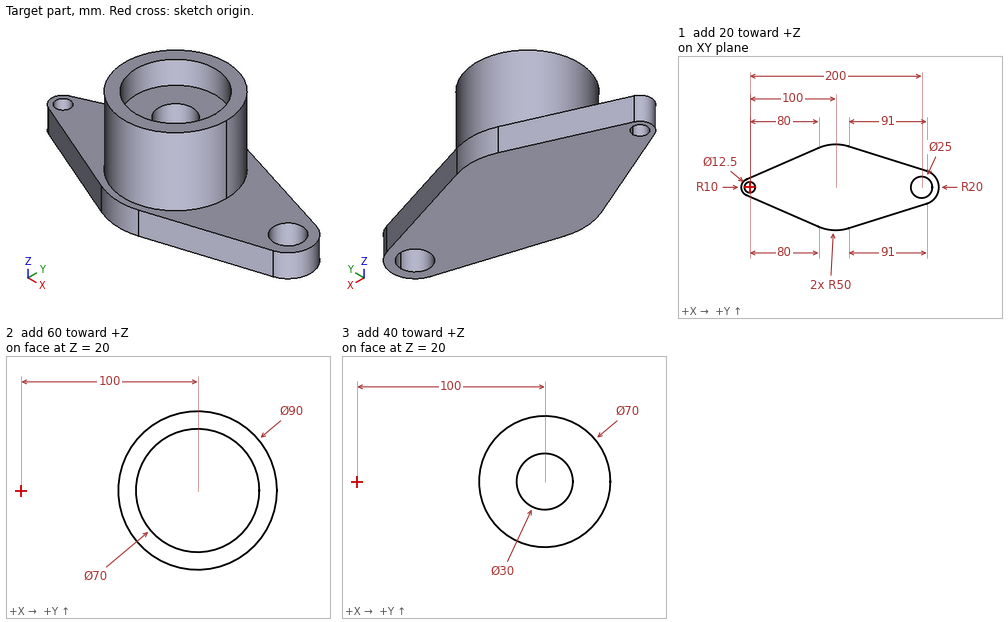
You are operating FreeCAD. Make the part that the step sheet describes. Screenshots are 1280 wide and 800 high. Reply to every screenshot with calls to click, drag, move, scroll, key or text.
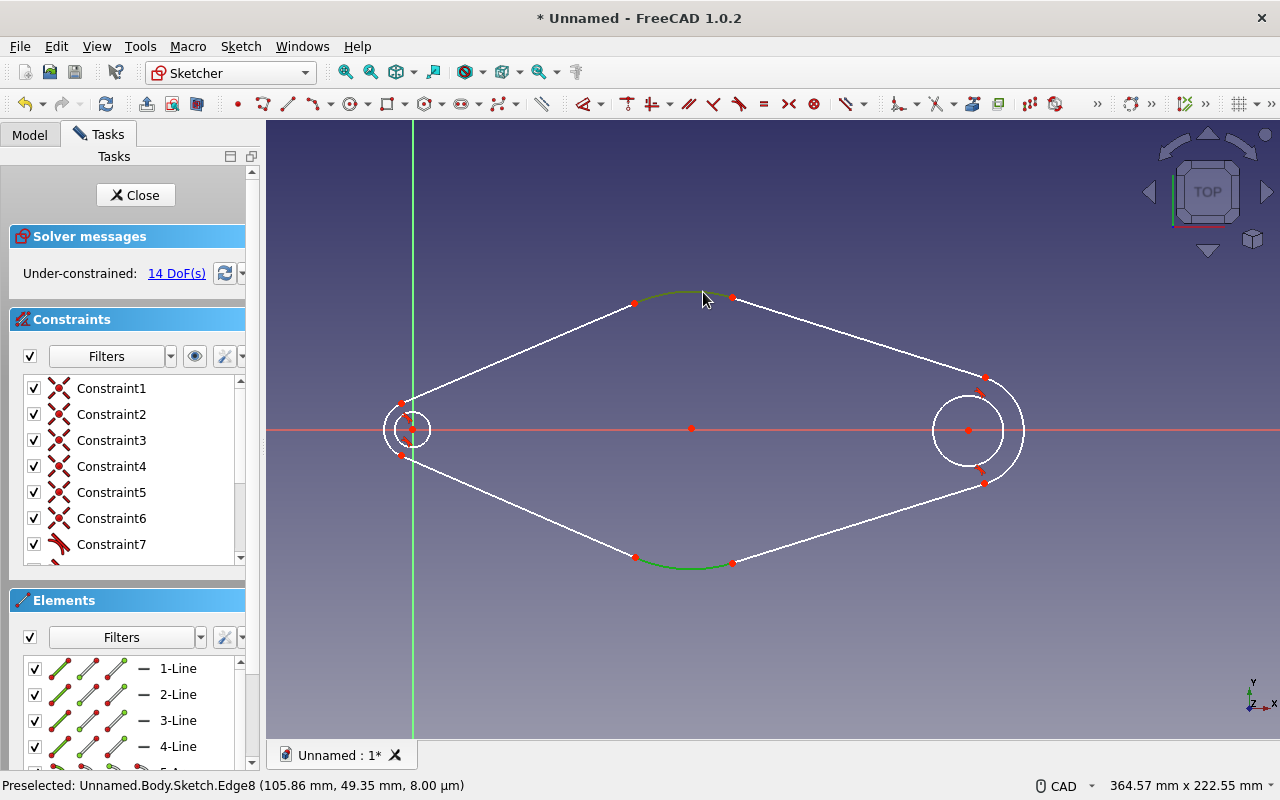
click(764, 104)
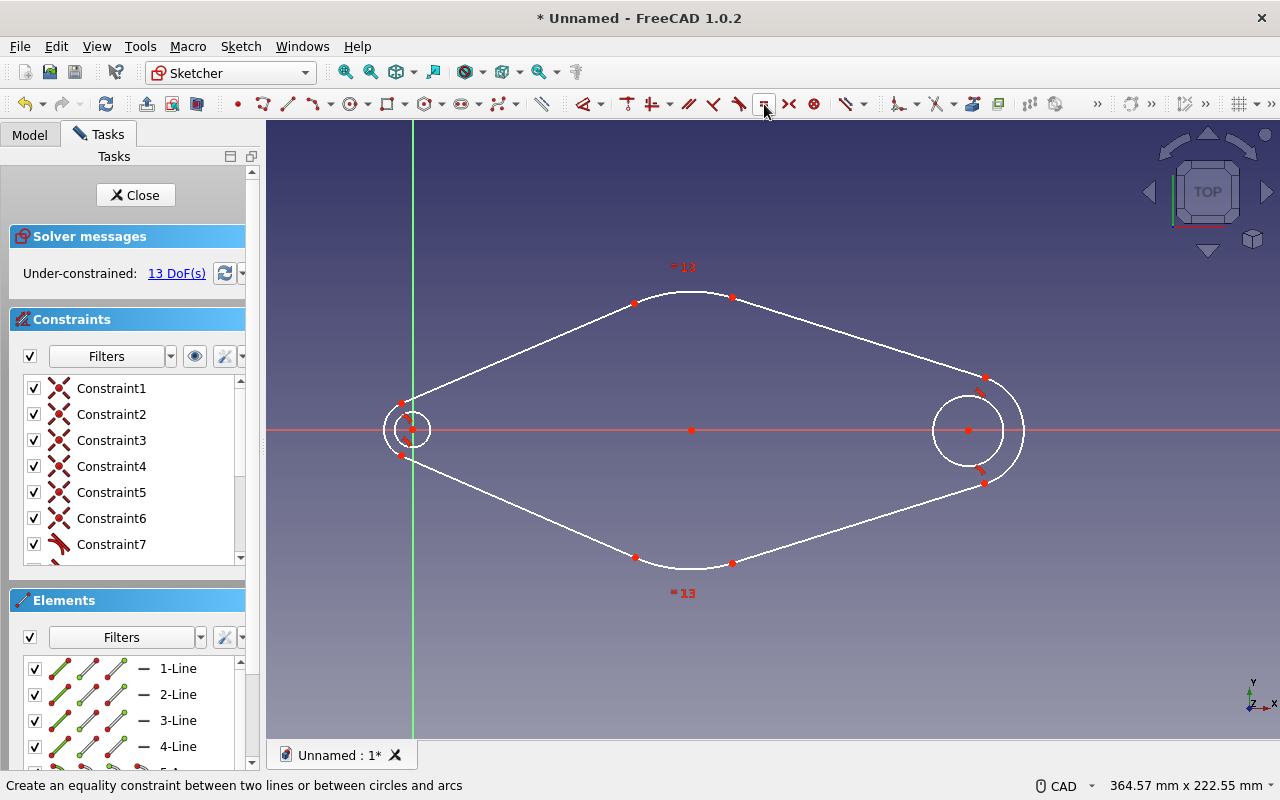
click(691, 431)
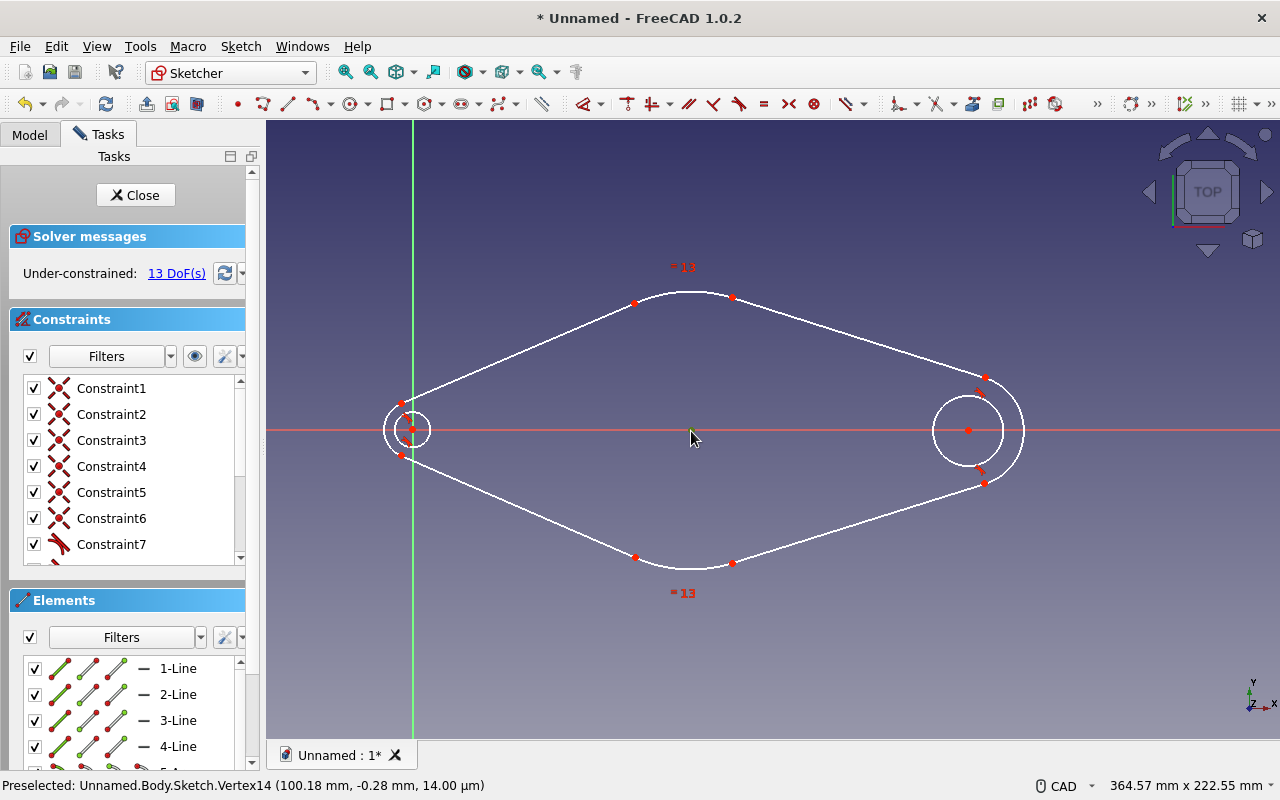
click(353, 430)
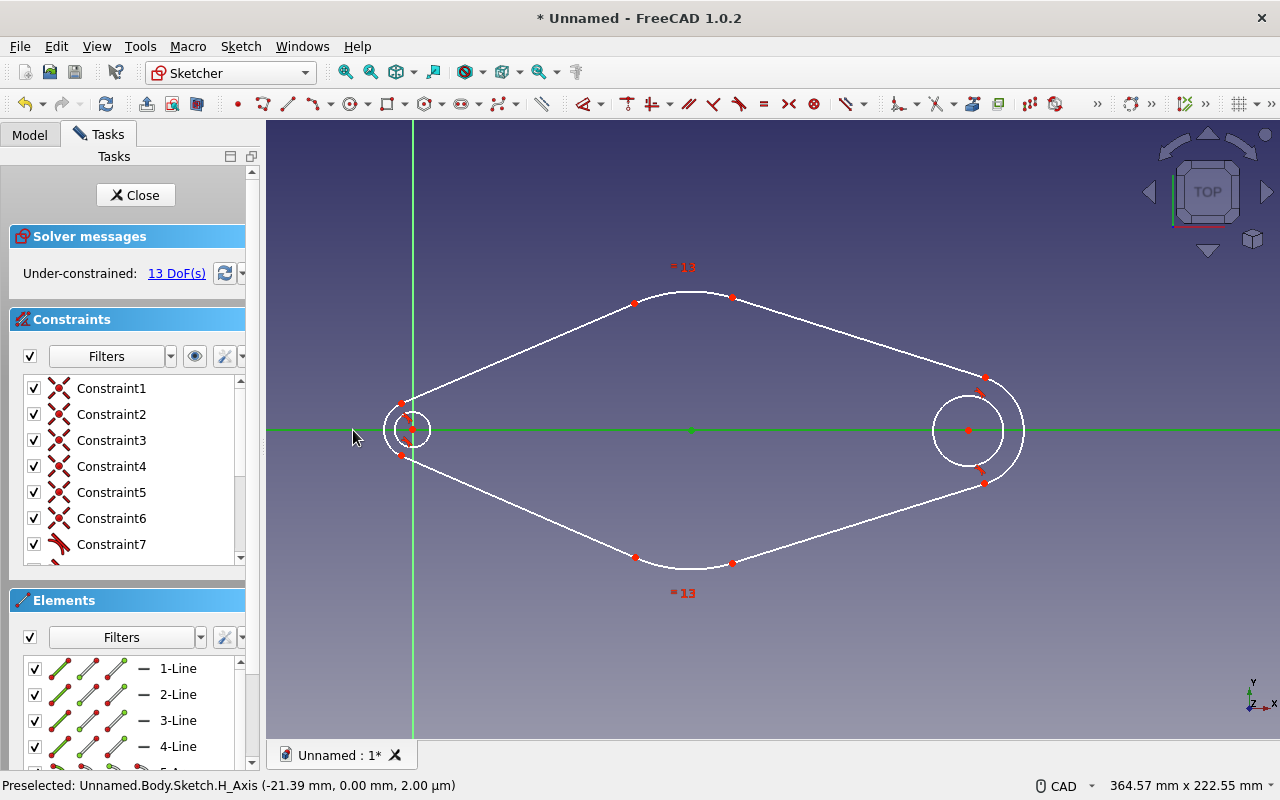
click(627, 104)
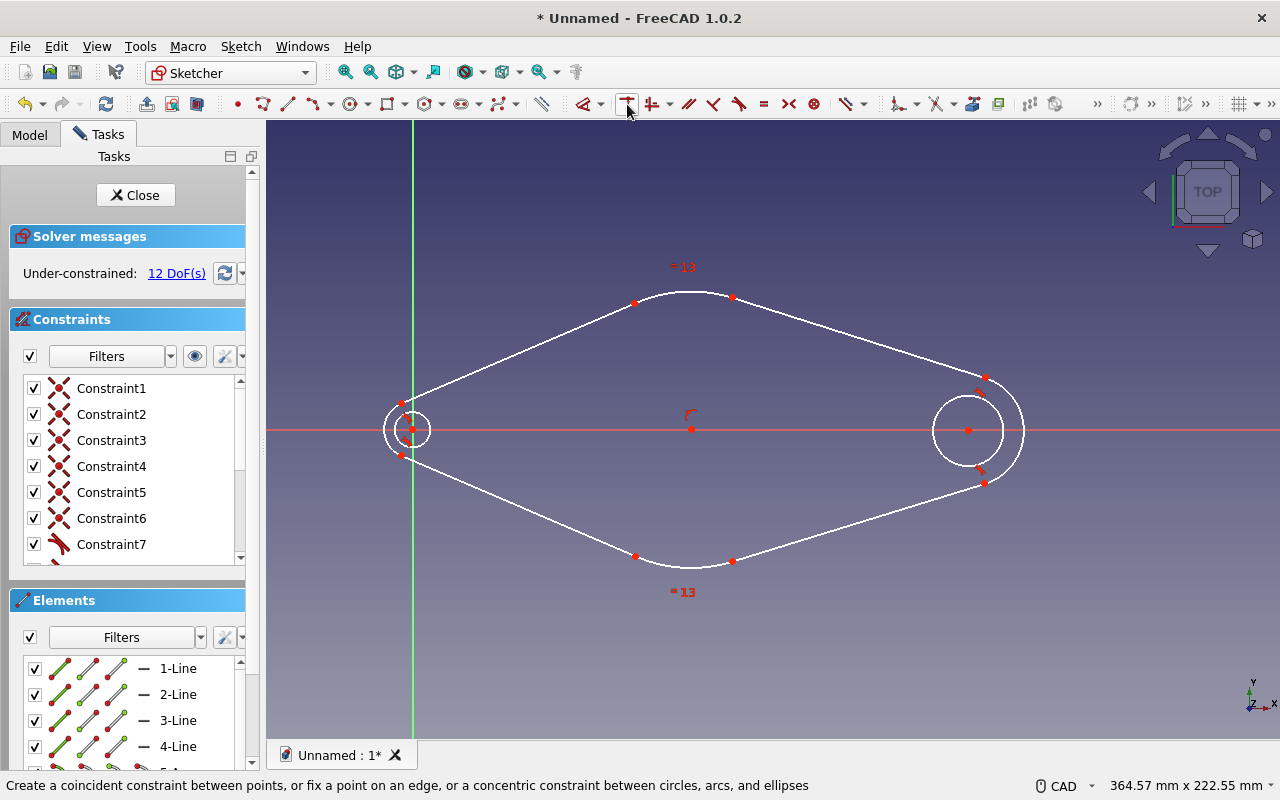
click(968, 431)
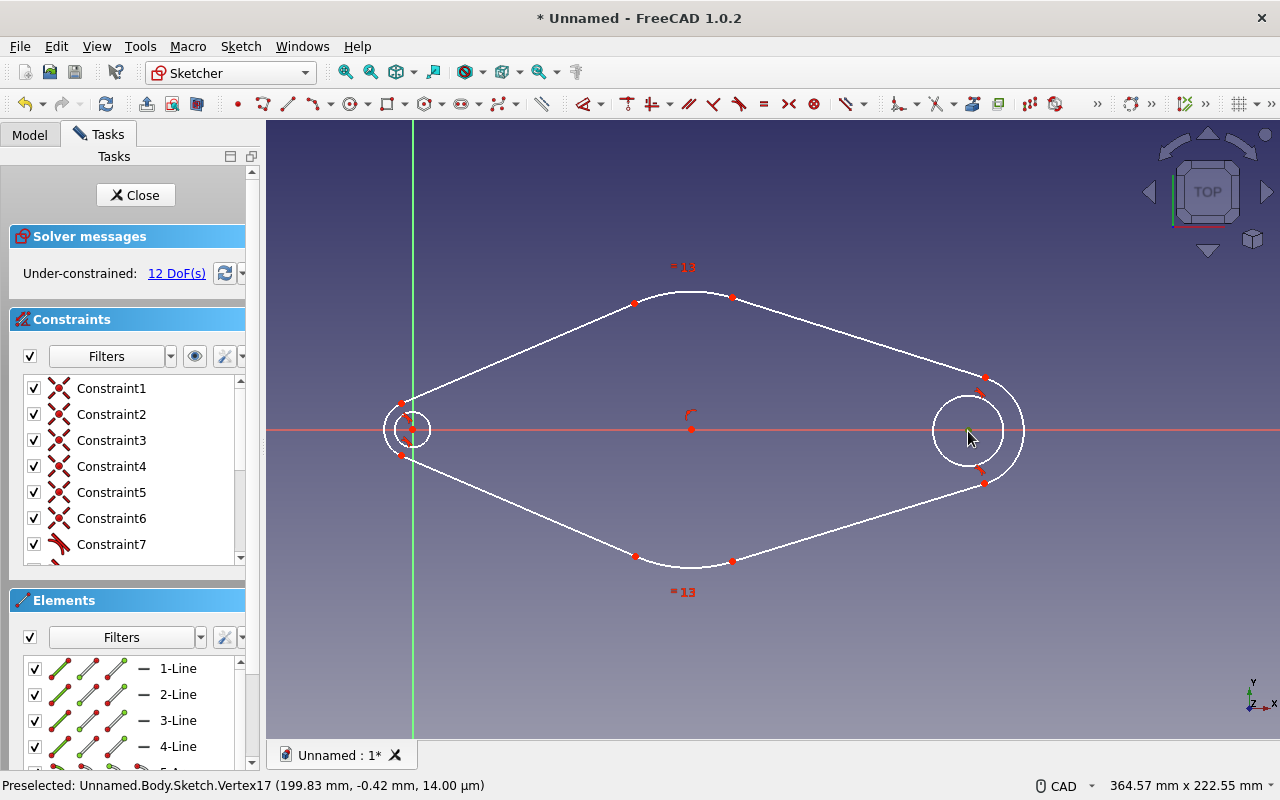
click(353, 430)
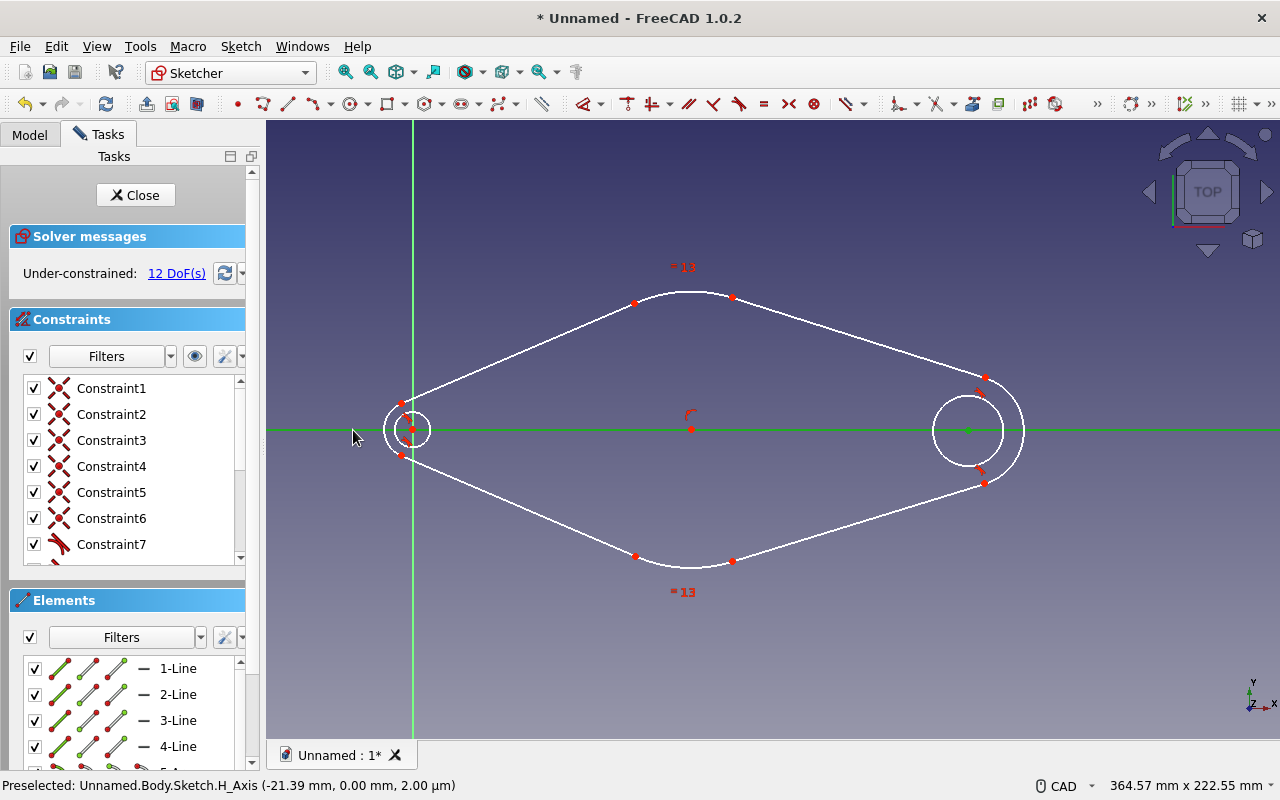
click(627, 104)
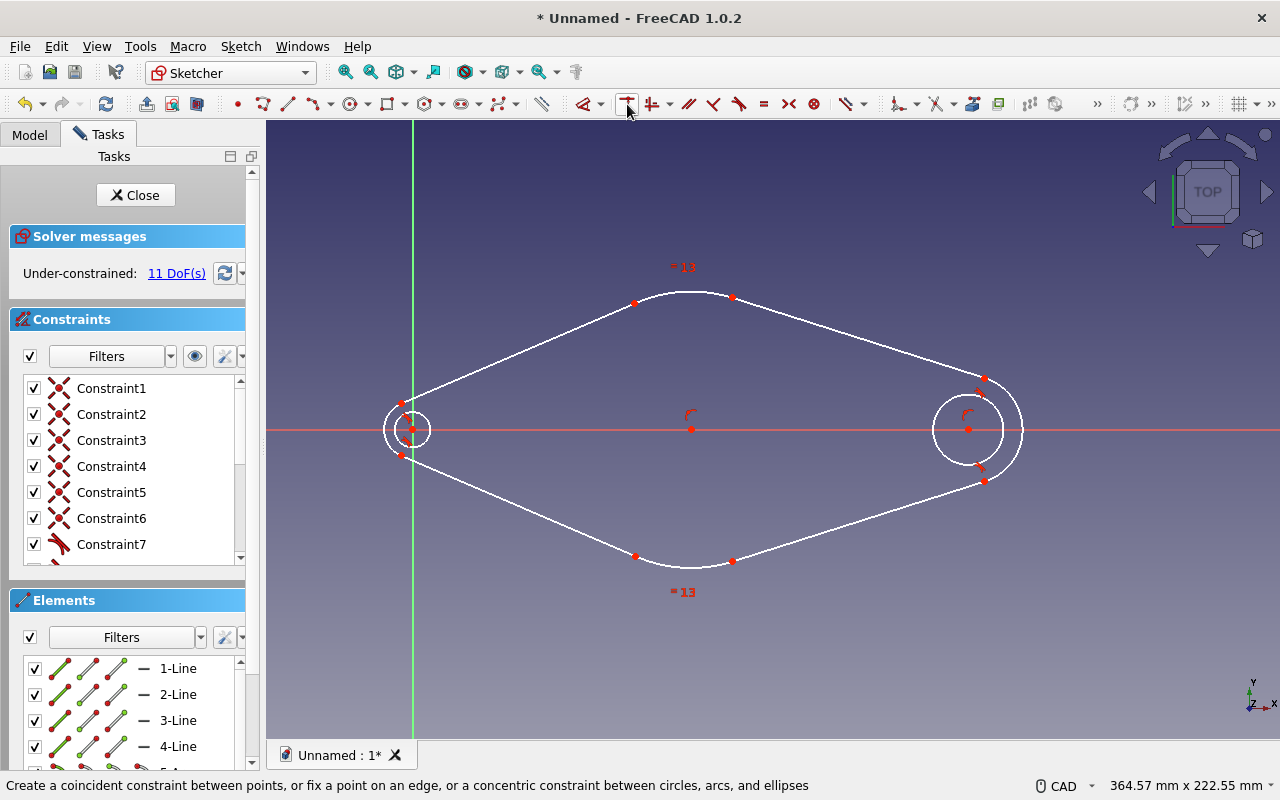
click(582, 104)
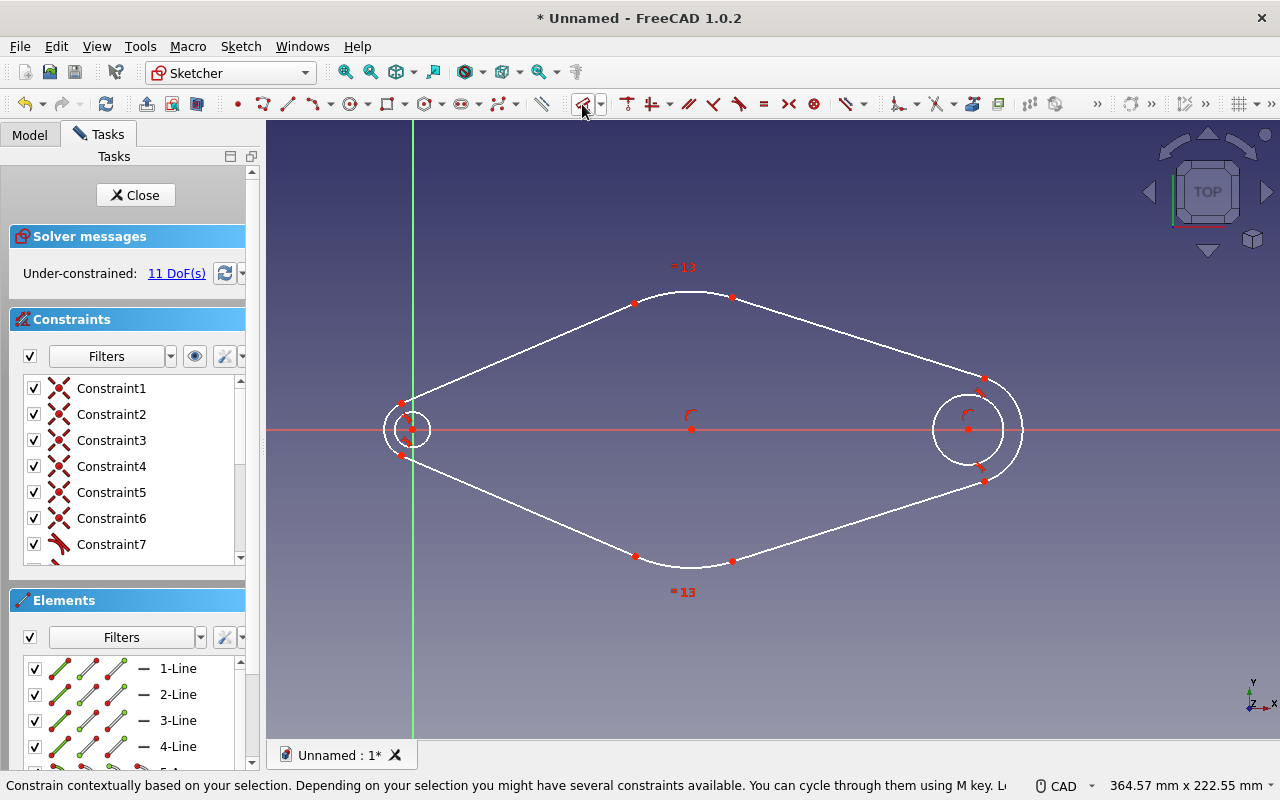
scroll(387, 417, up, 2)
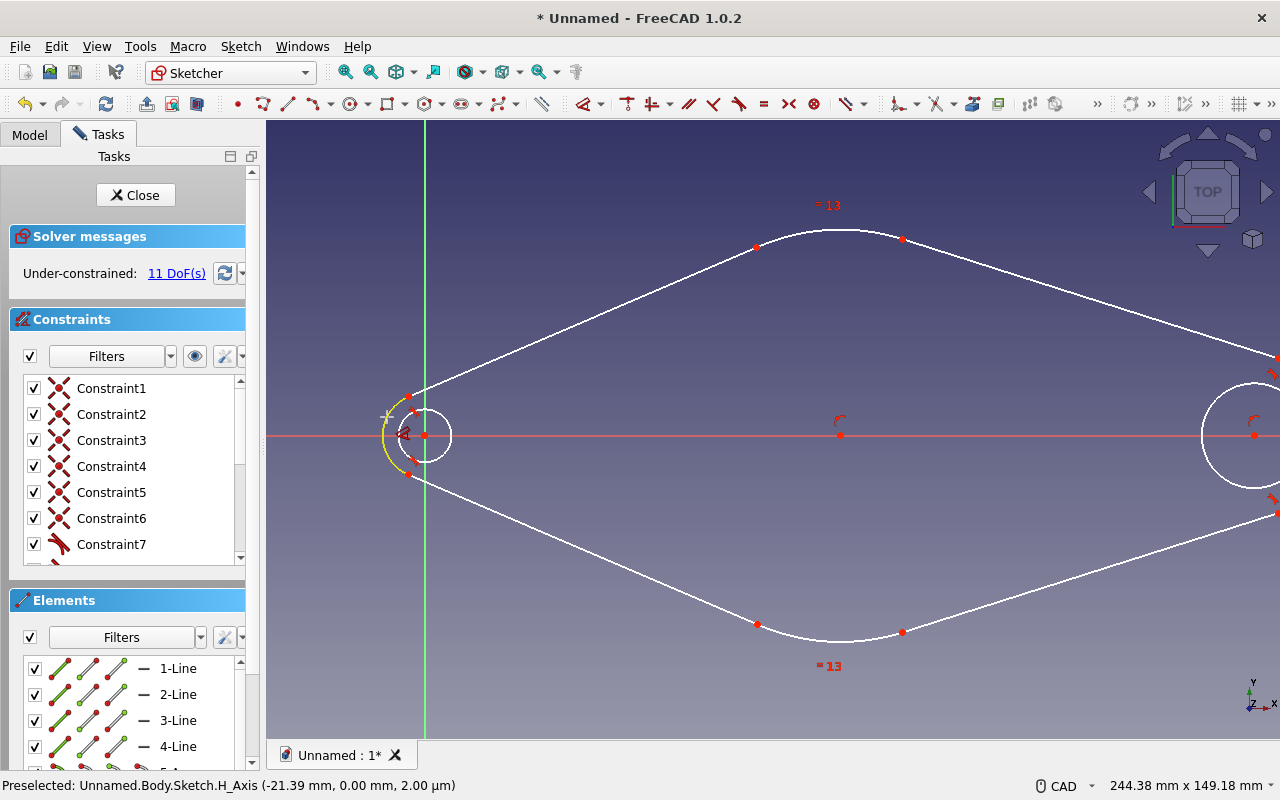
click(387, 417)
click(358, 403)